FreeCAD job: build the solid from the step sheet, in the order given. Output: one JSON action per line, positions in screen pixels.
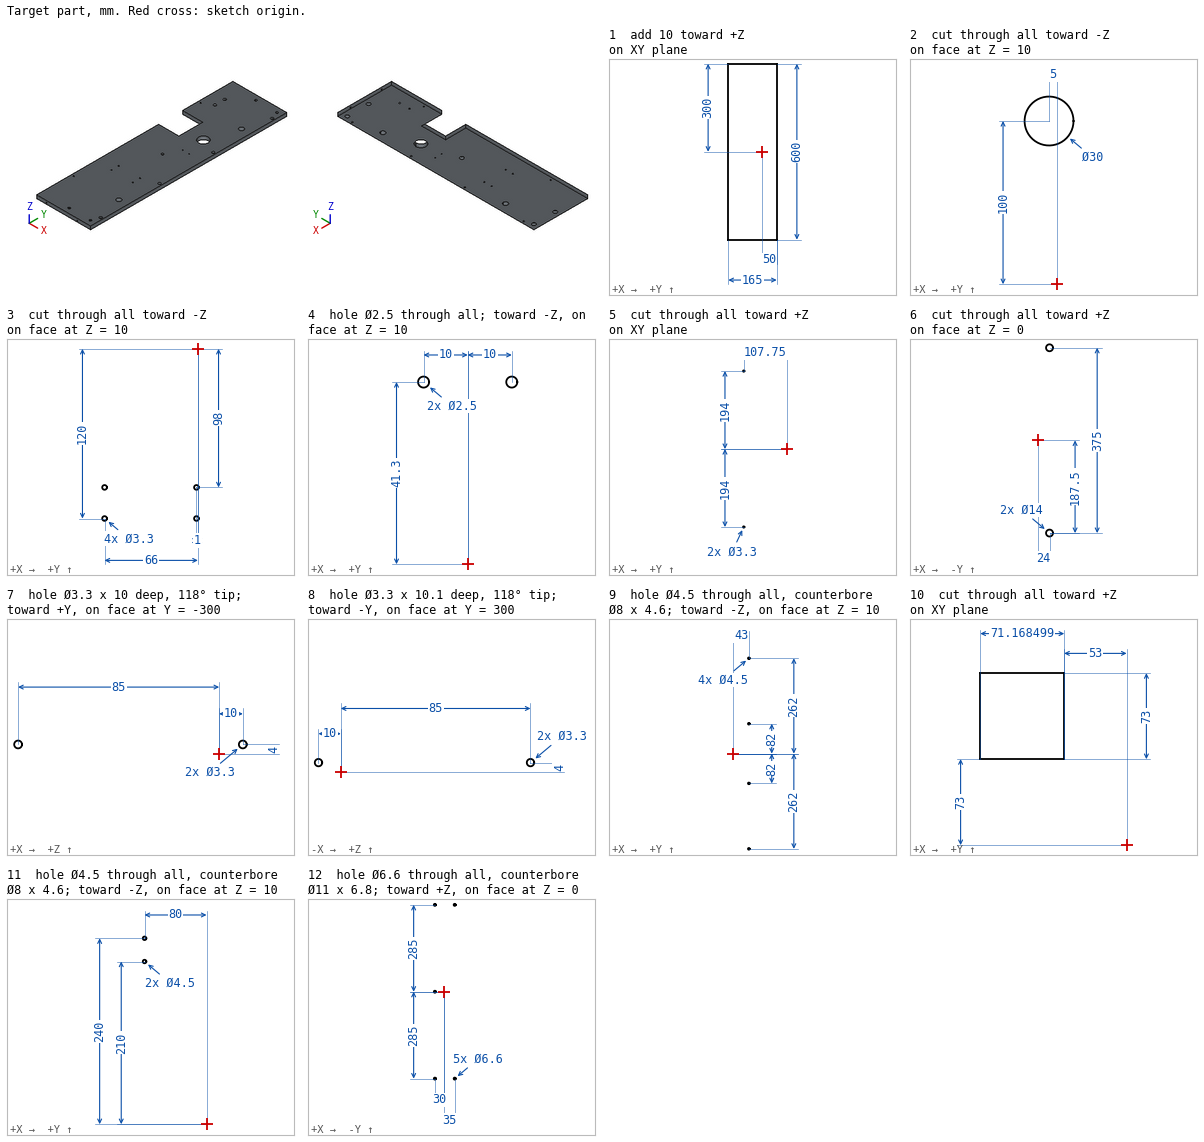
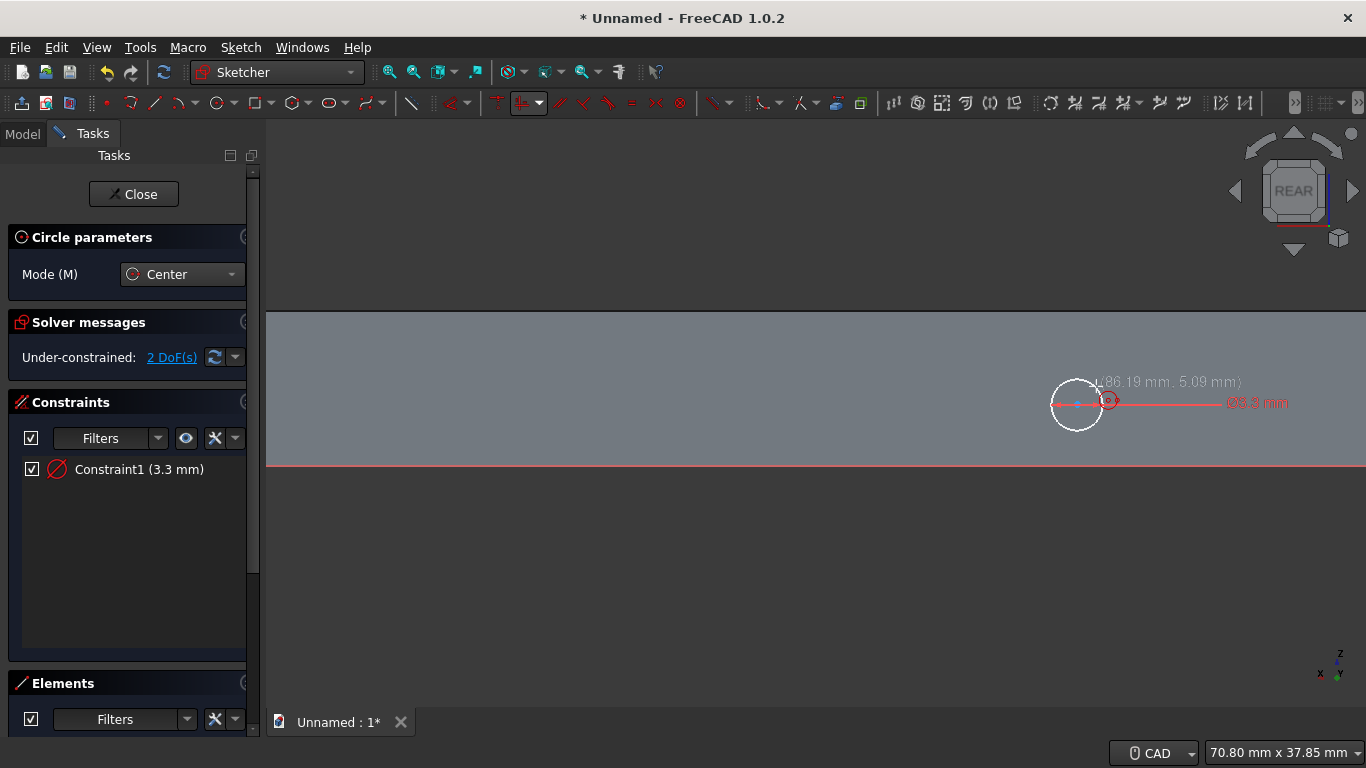
{"action": "scroll", "coordinate": [1080, 405], "scroll_direction": "down", "scroll_amount": 4}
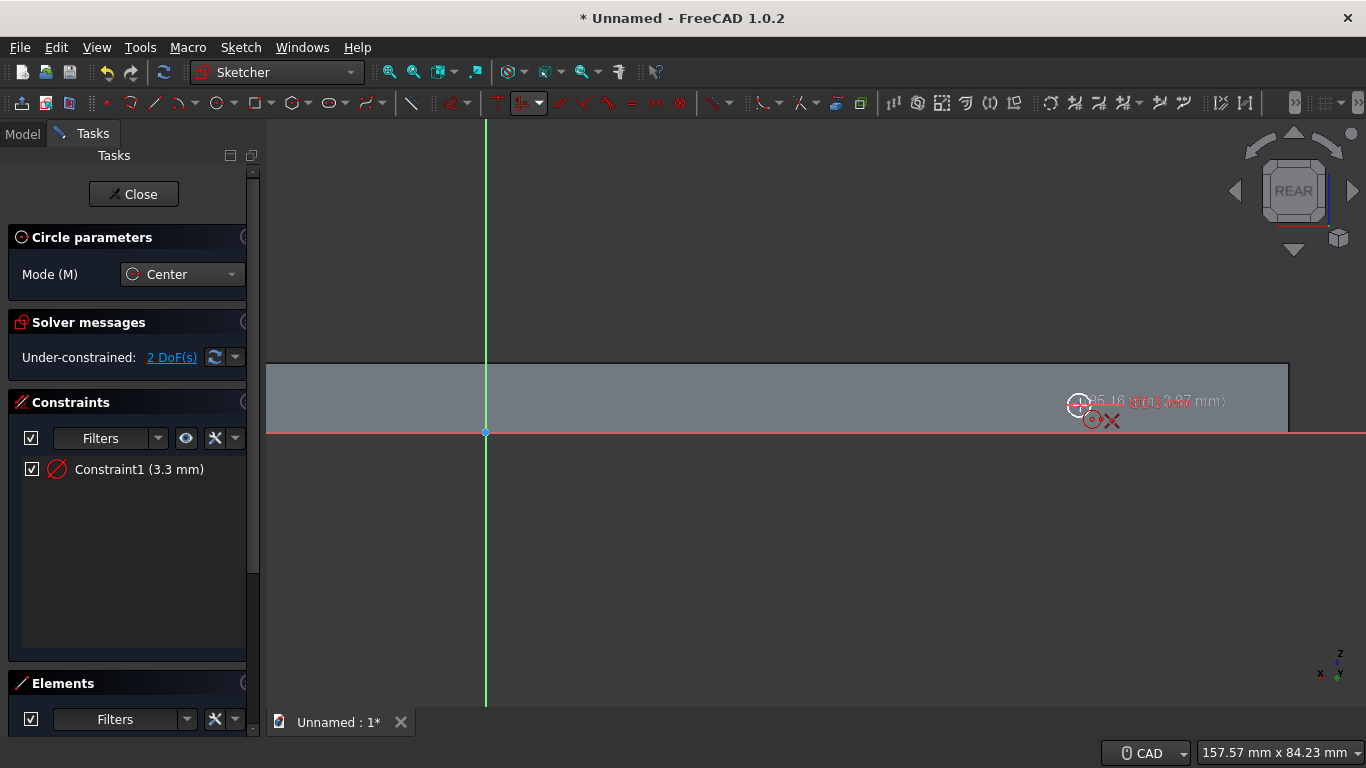
{"action": "scroll", "coordinate": [416, 405], "scroll_direction": "up", "scroll_amount": 4}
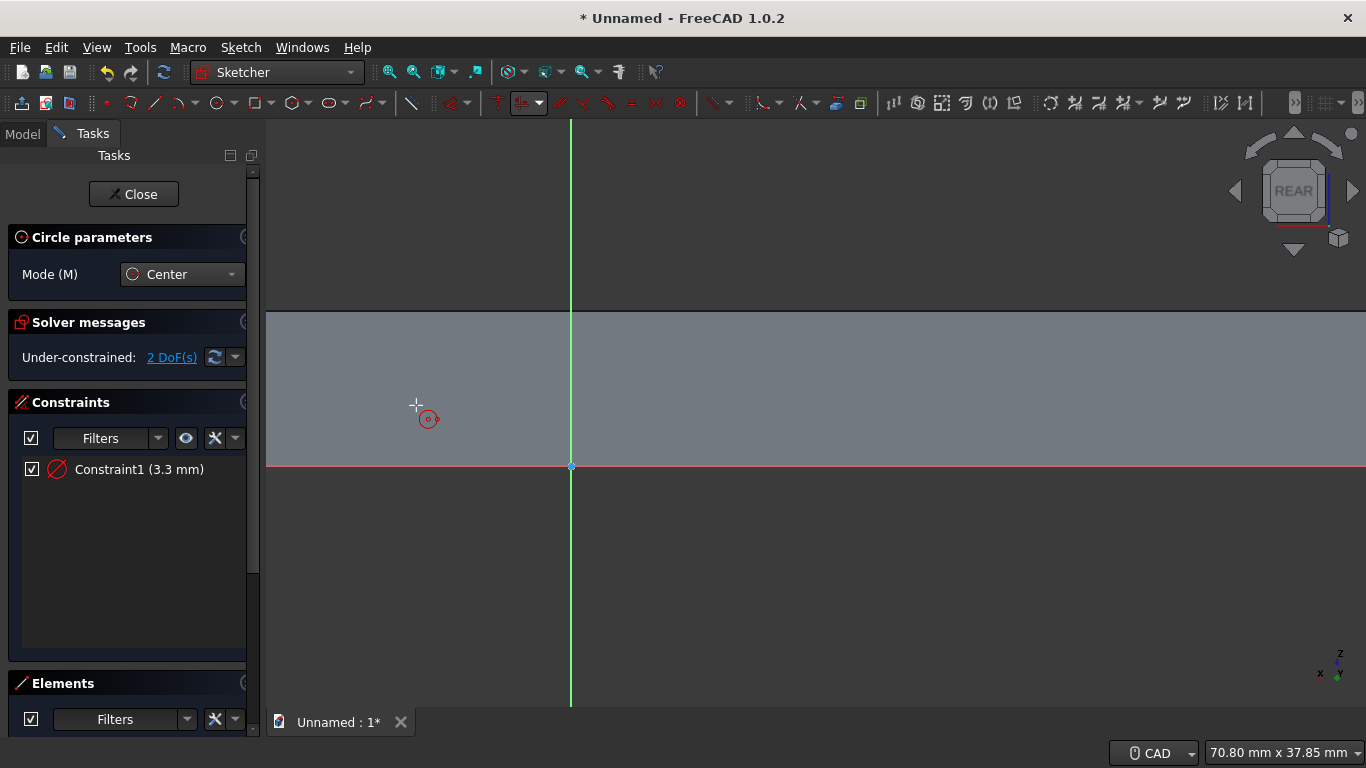
{"action": "left_click", "coordinate": [416, 404]}
{"action": "mouse_move", "coordinate": [434, 386]}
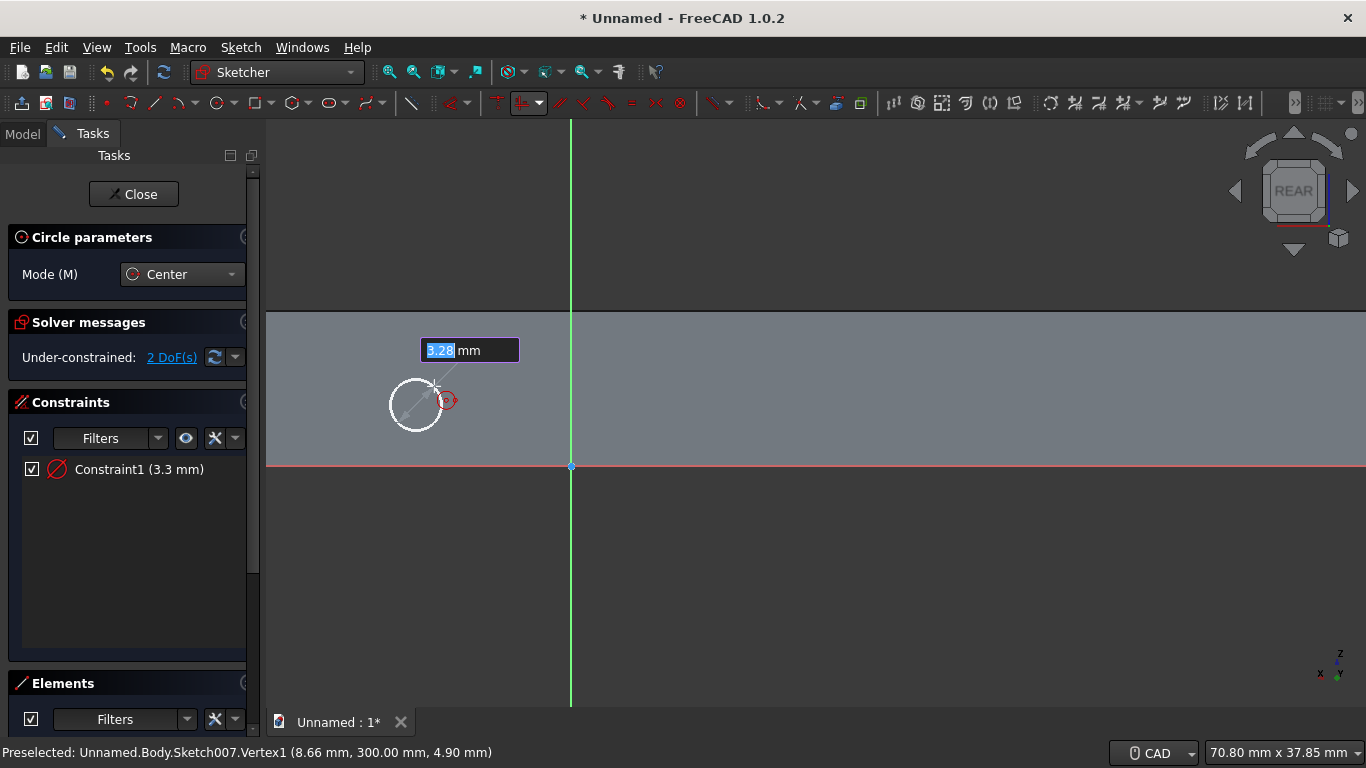
{"action": "type", "text": "3.3"}
{"action": "key", "text": "Return"}
{"action": "key", "text": "Escape"}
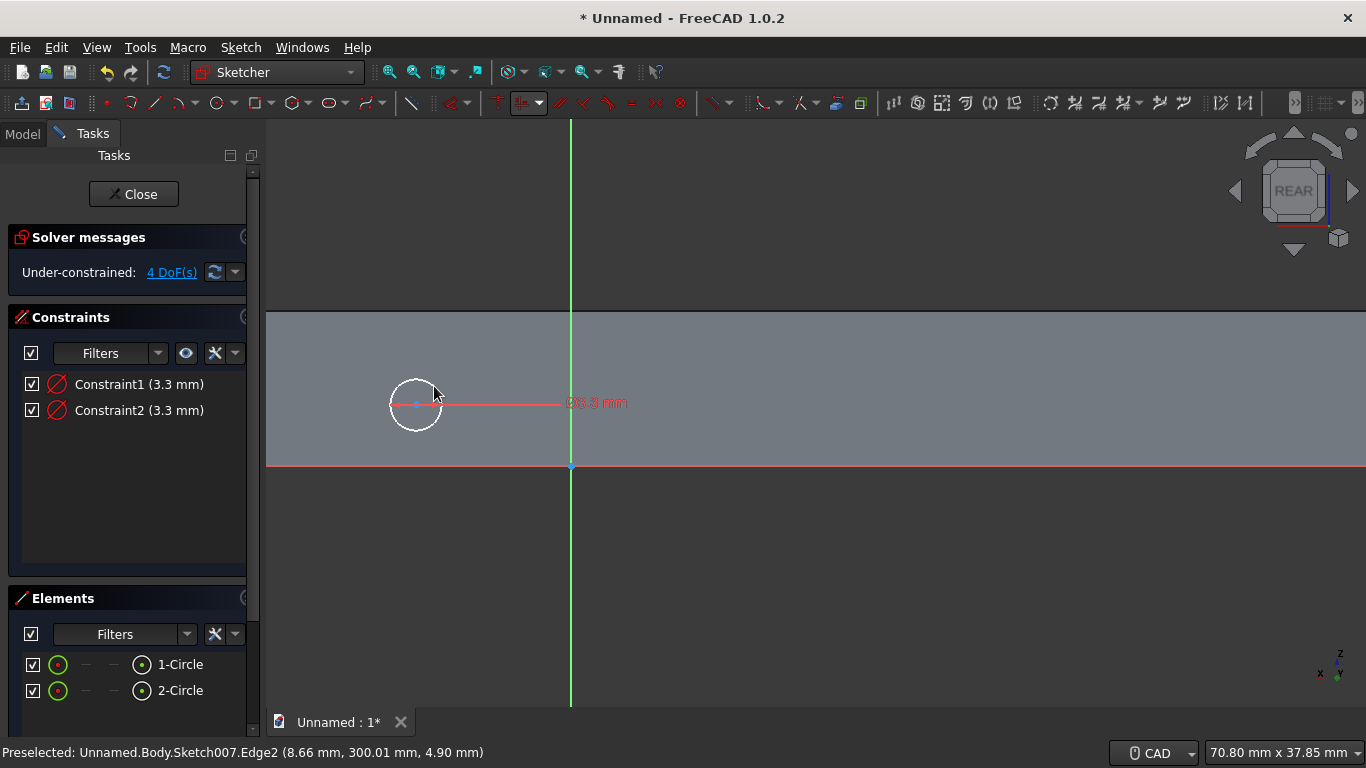
{"action": "scroll", "coordinate": [416, 405], "scroll_direction": "down", "scroll_amount": 4}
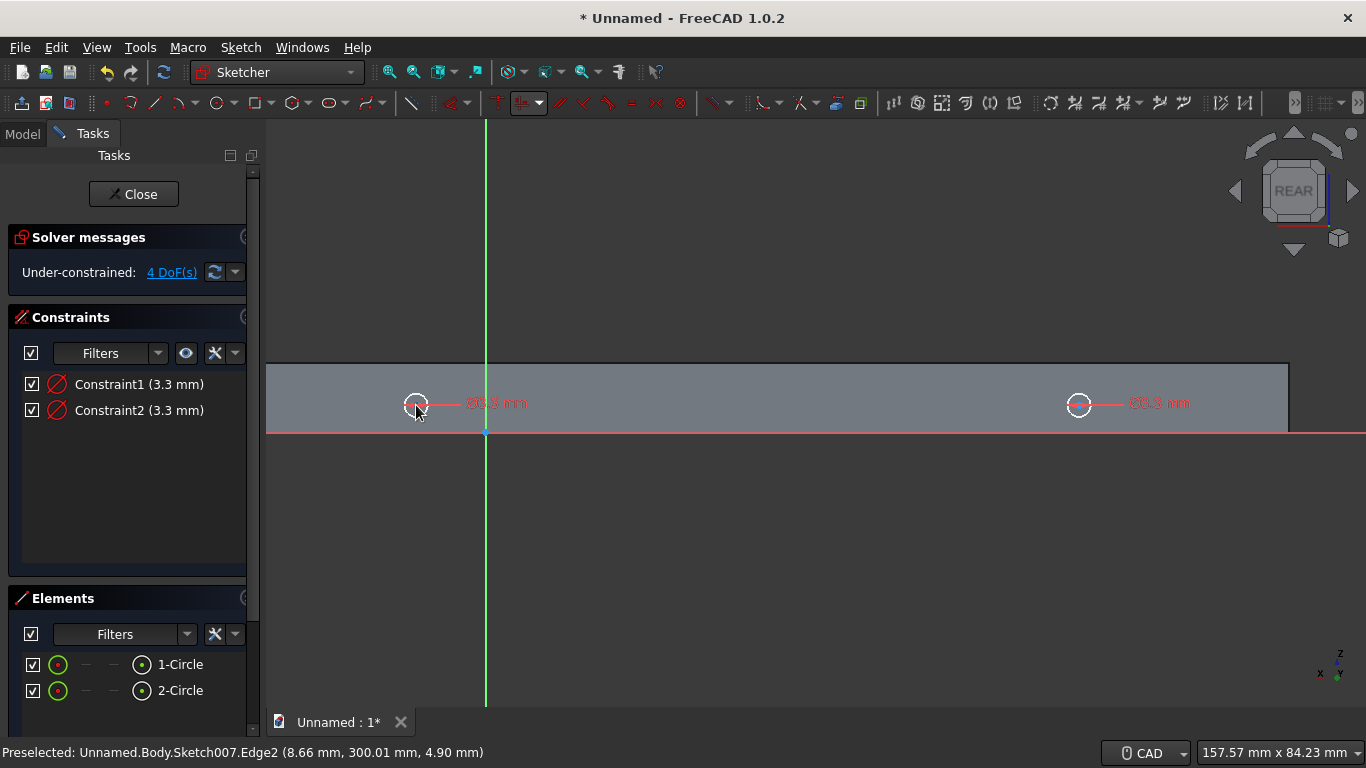
{"action": "left_click", "coordinate": [1079, 405]}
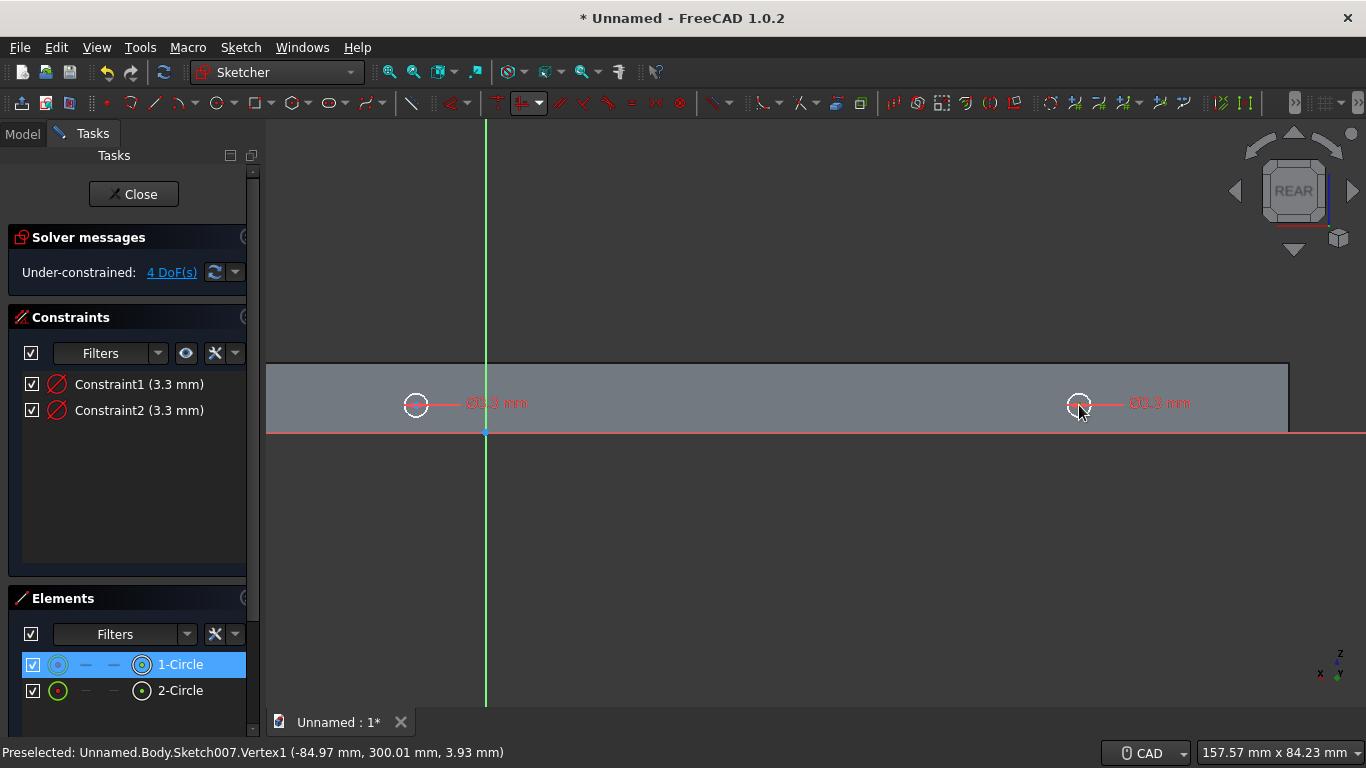
{"action": "left_click", "coordinate": [416, 405]}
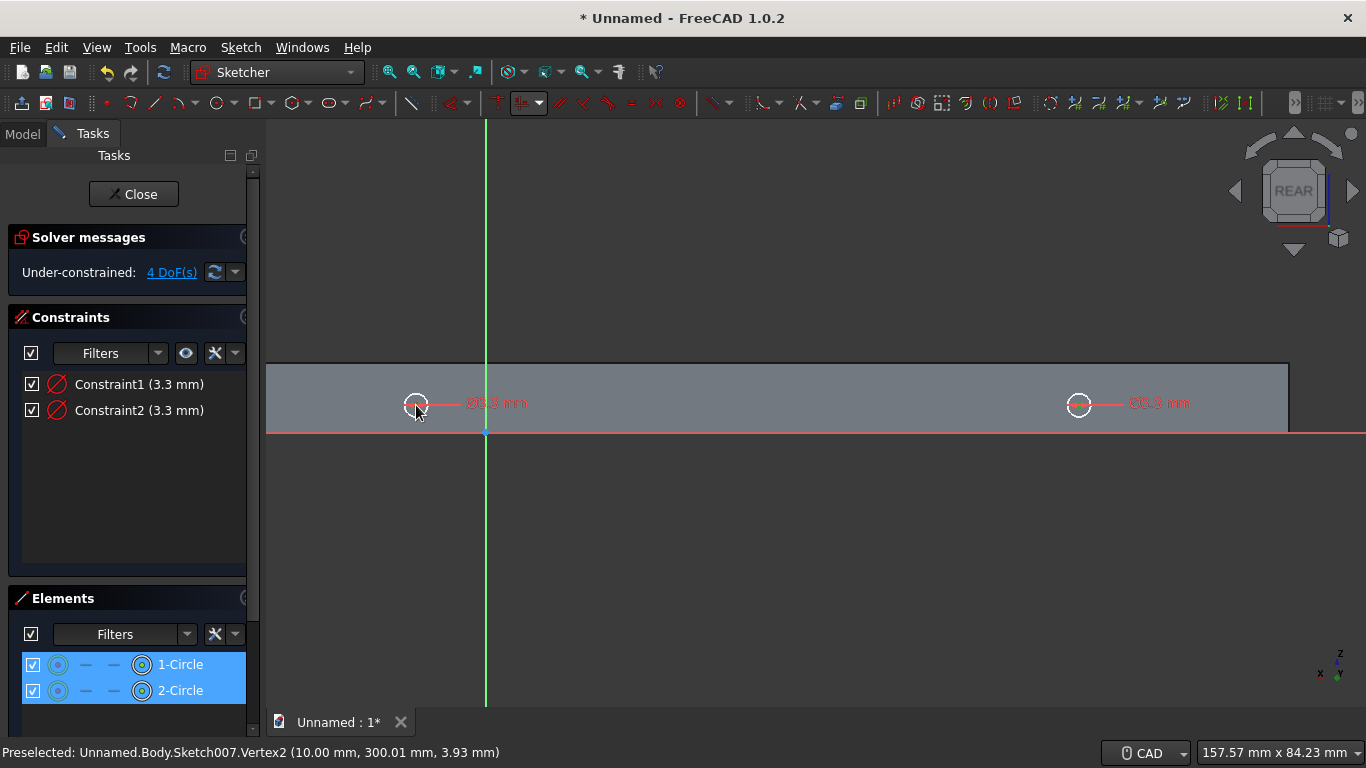
{"action": "left_click", "coordinate": [542, 104]}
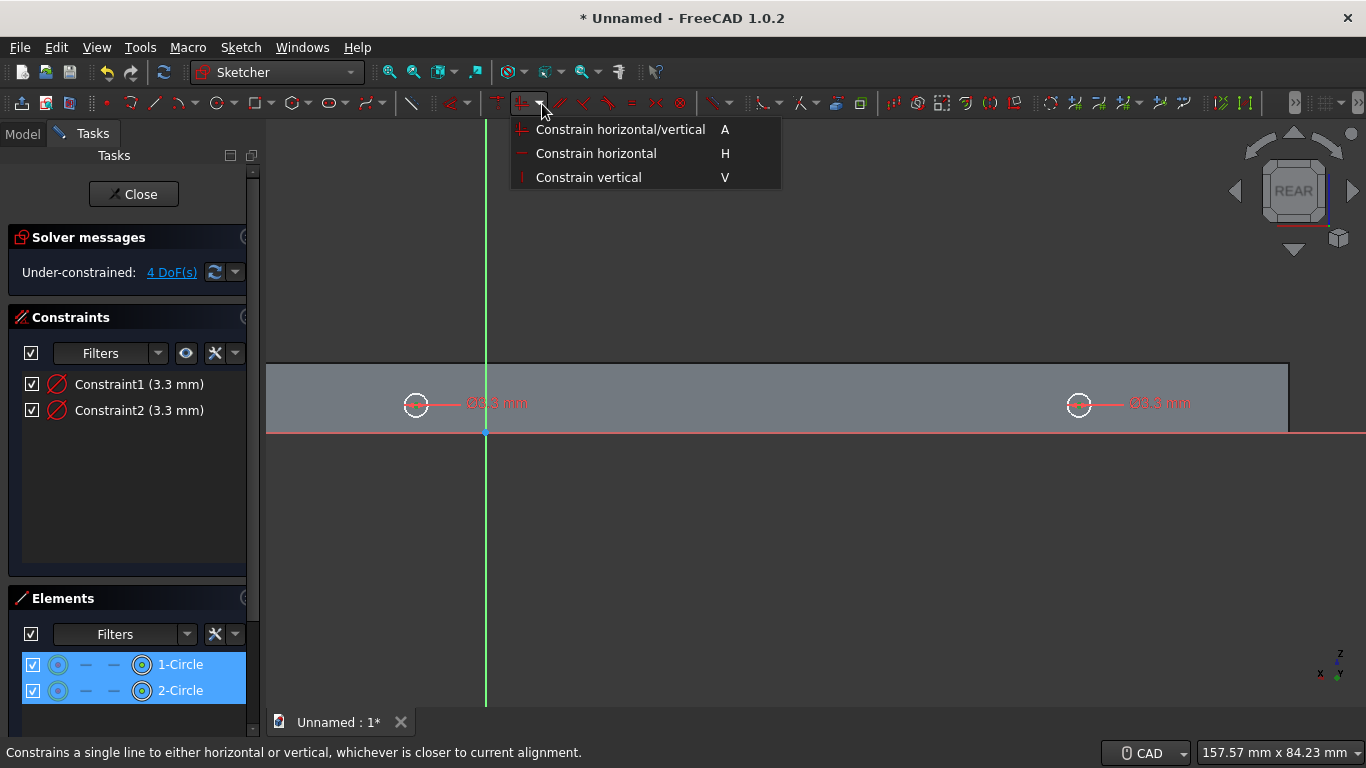
{"action": "left_click", "coordinate": [646, 153]}